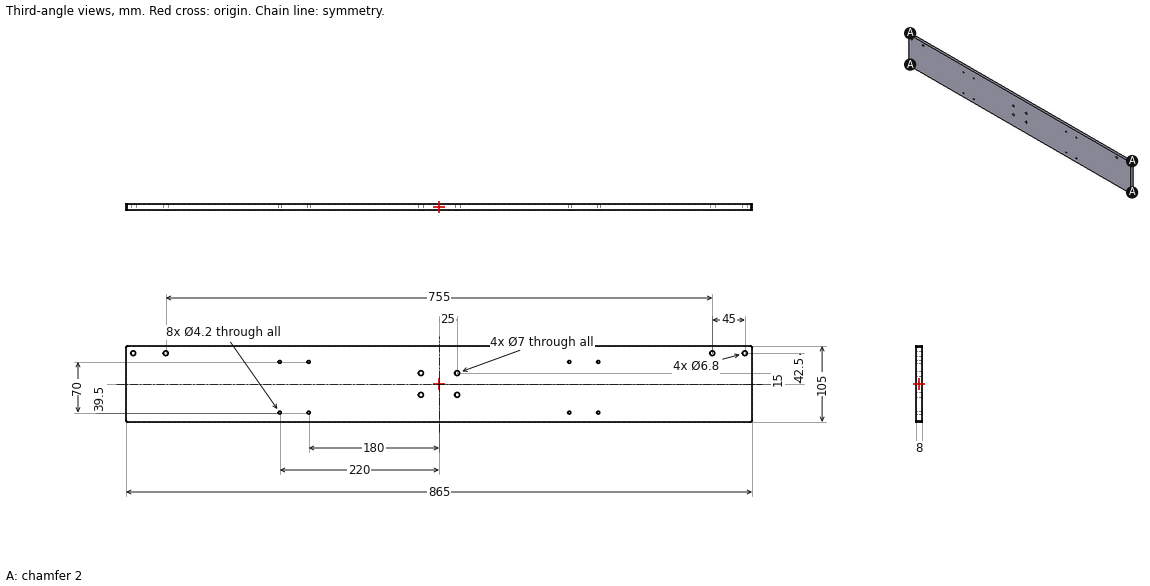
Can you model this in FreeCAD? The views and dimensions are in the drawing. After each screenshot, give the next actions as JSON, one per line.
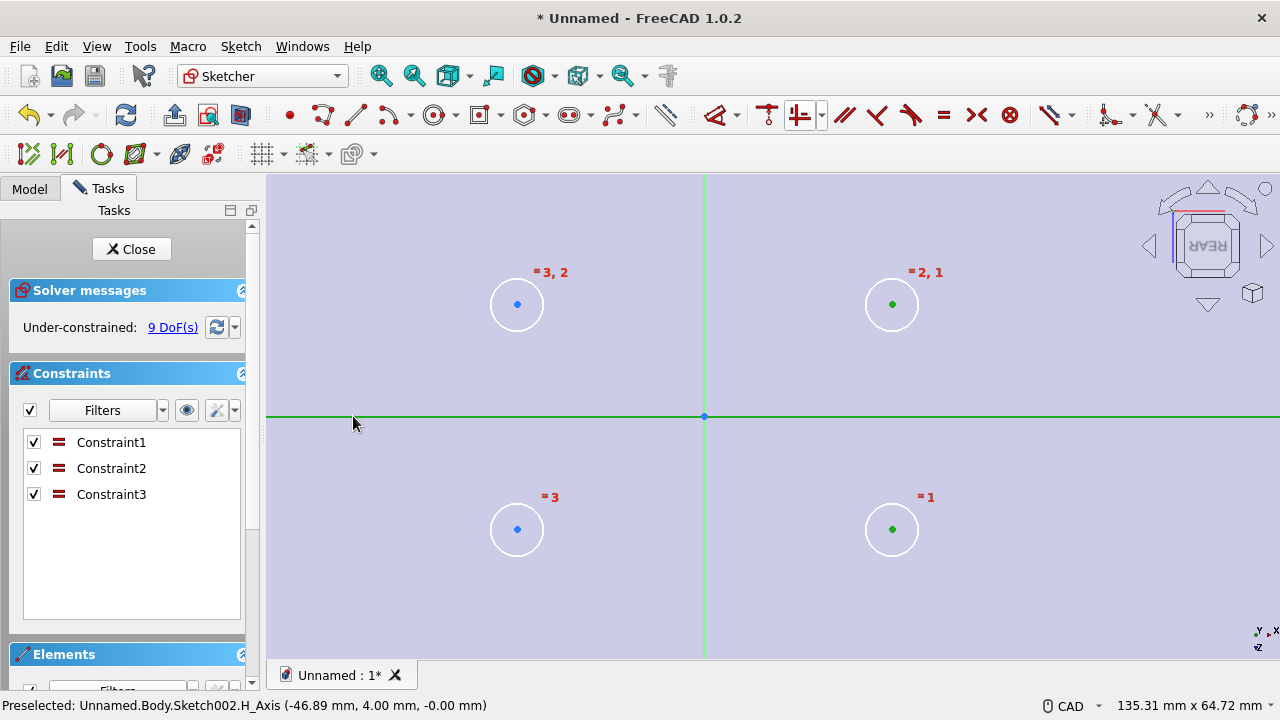
{"action": "key", "text": "s"}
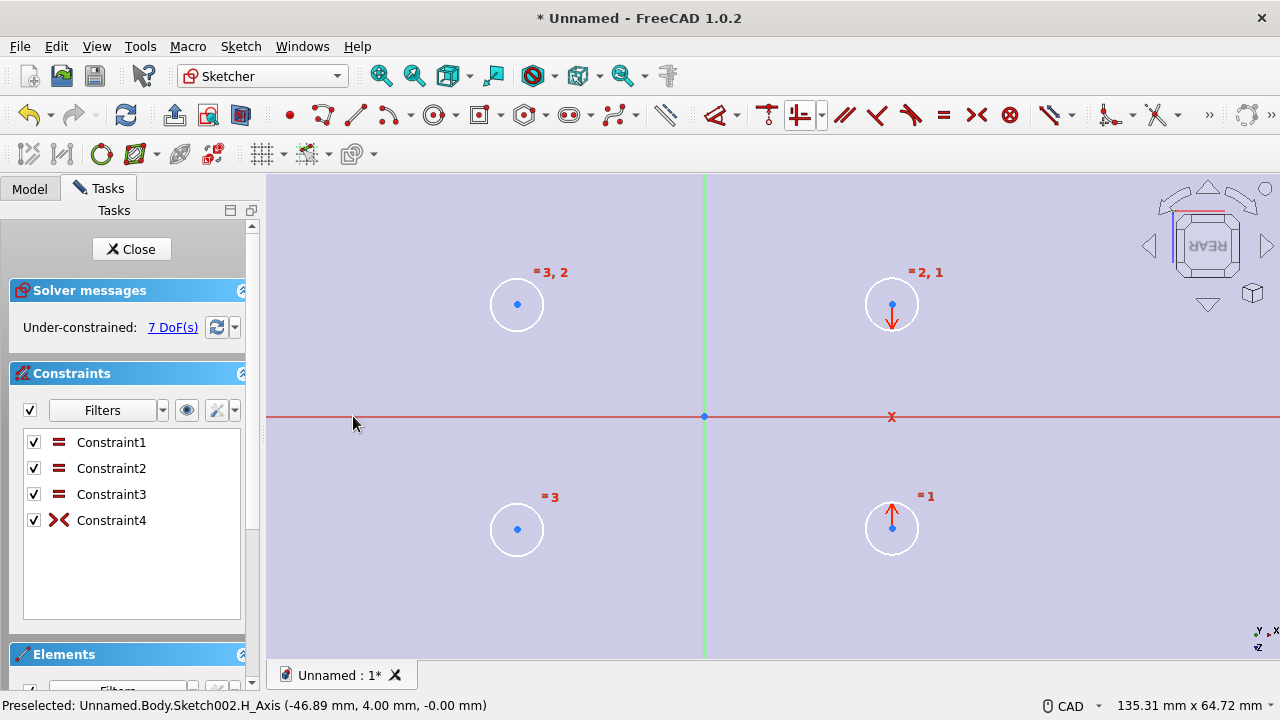
{"action": "left_click", "coordinate": [892, 304]}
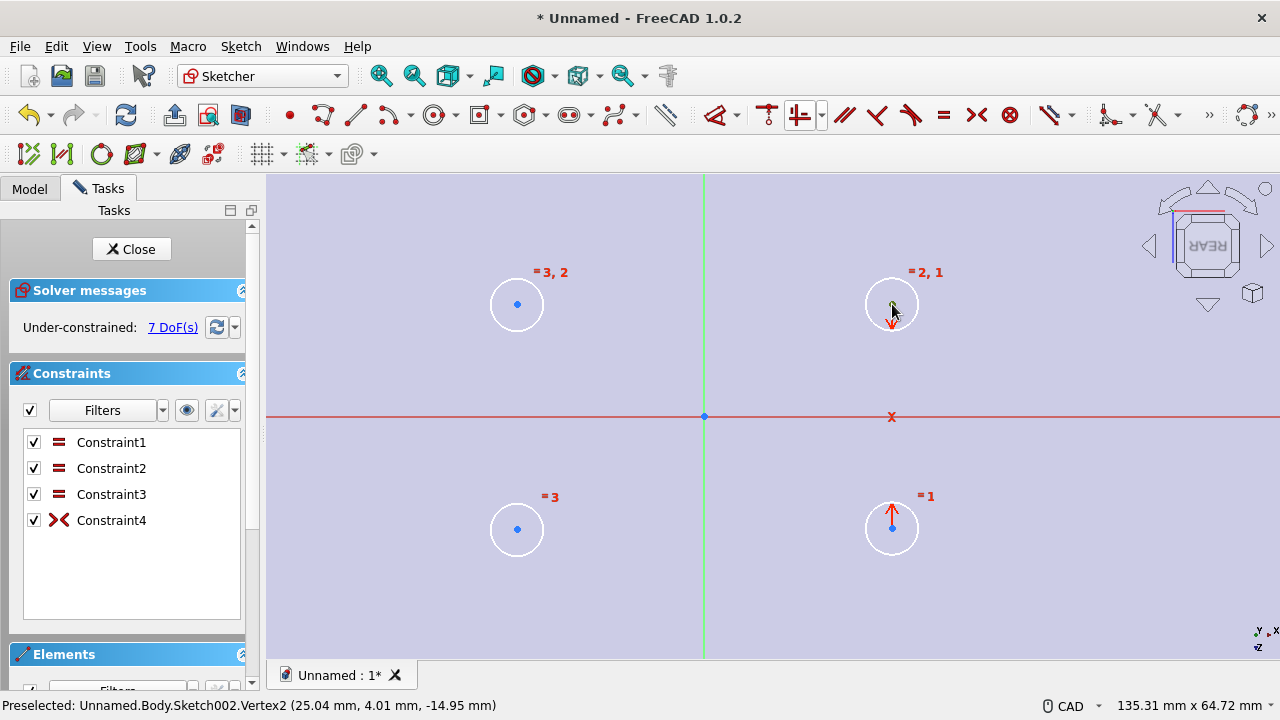
{"action": "left_click", "coordinate": [517, 305]}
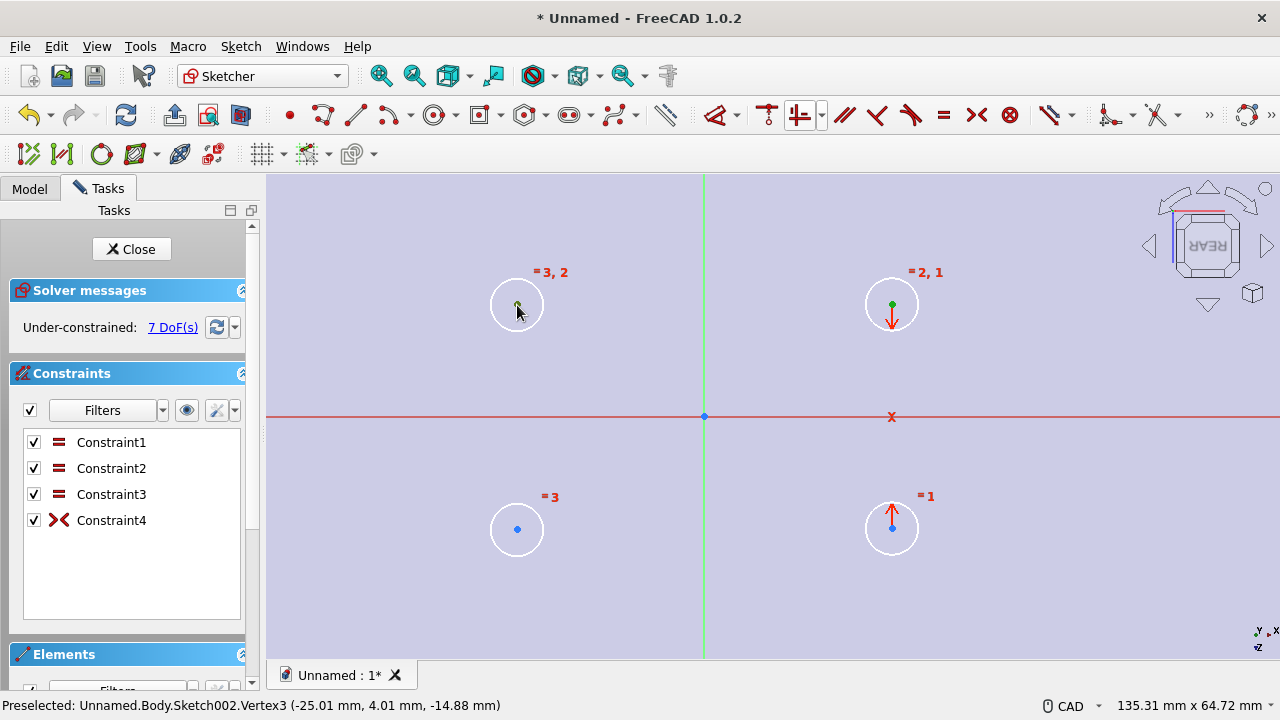
{"action": "left_click", "coordinate": [704, 600]}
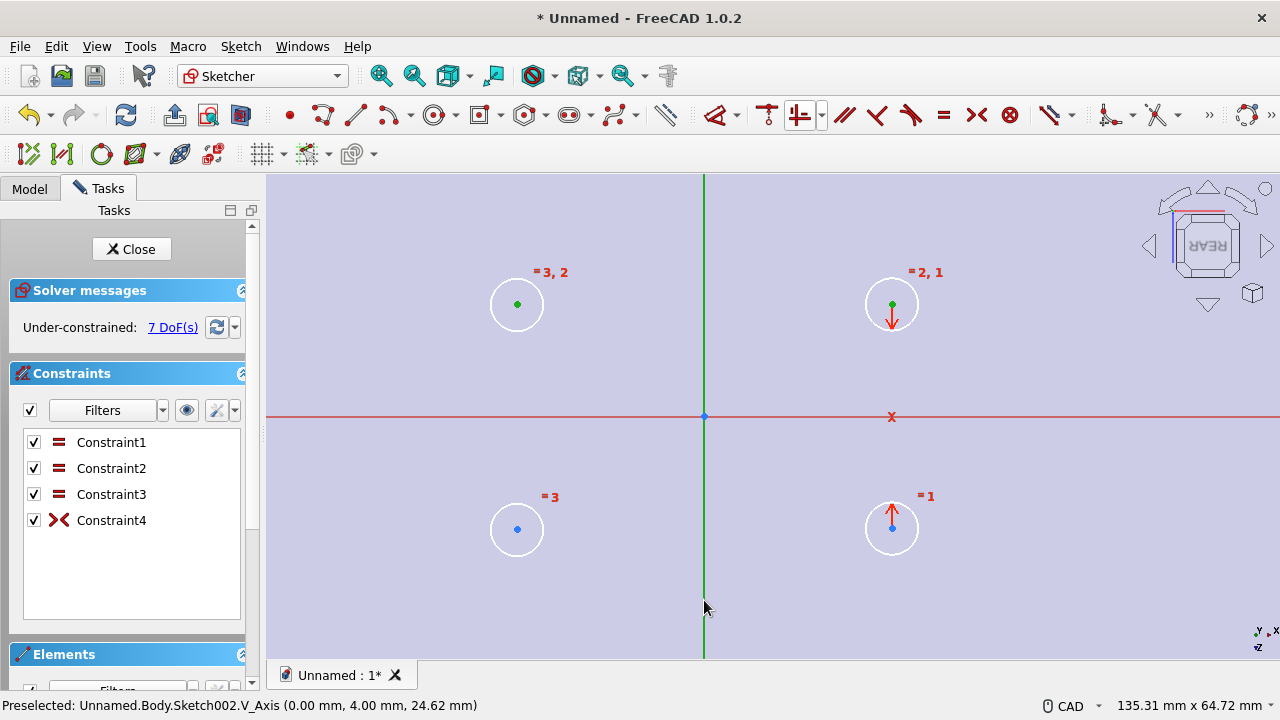
{"action": "key", "text": "s"}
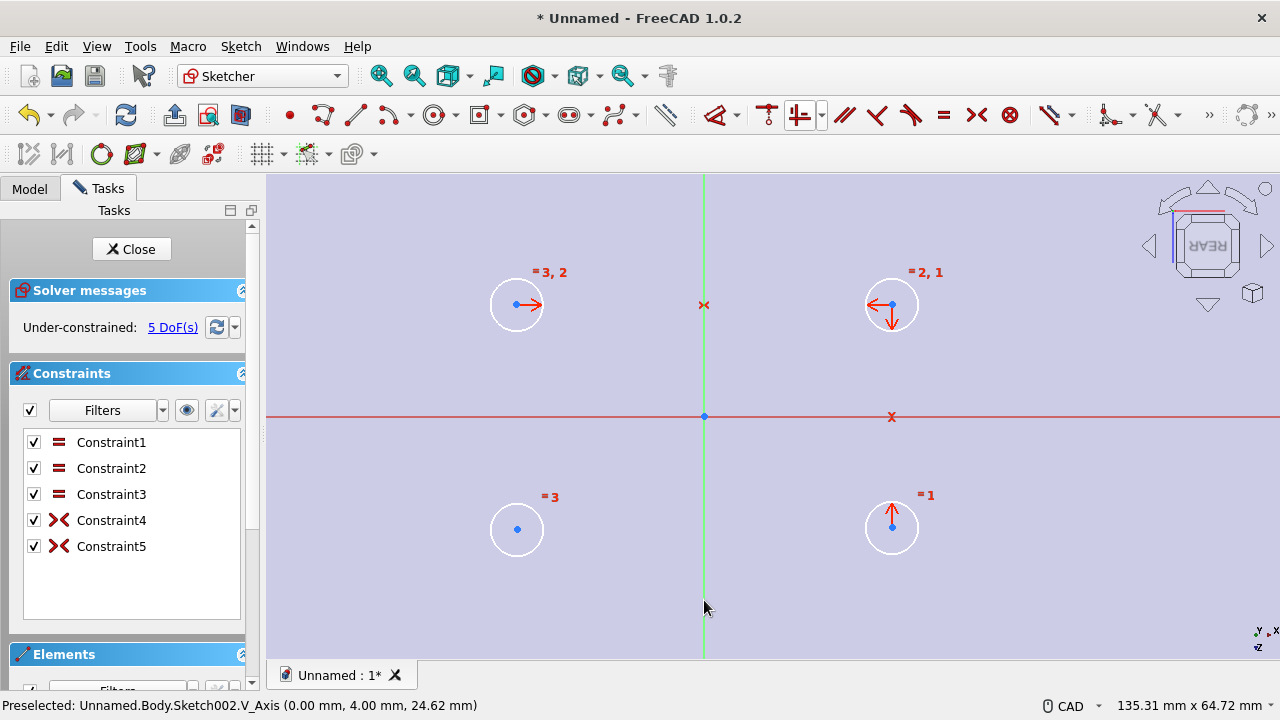
{"action": "left_click", "coordinate": [892, 528]}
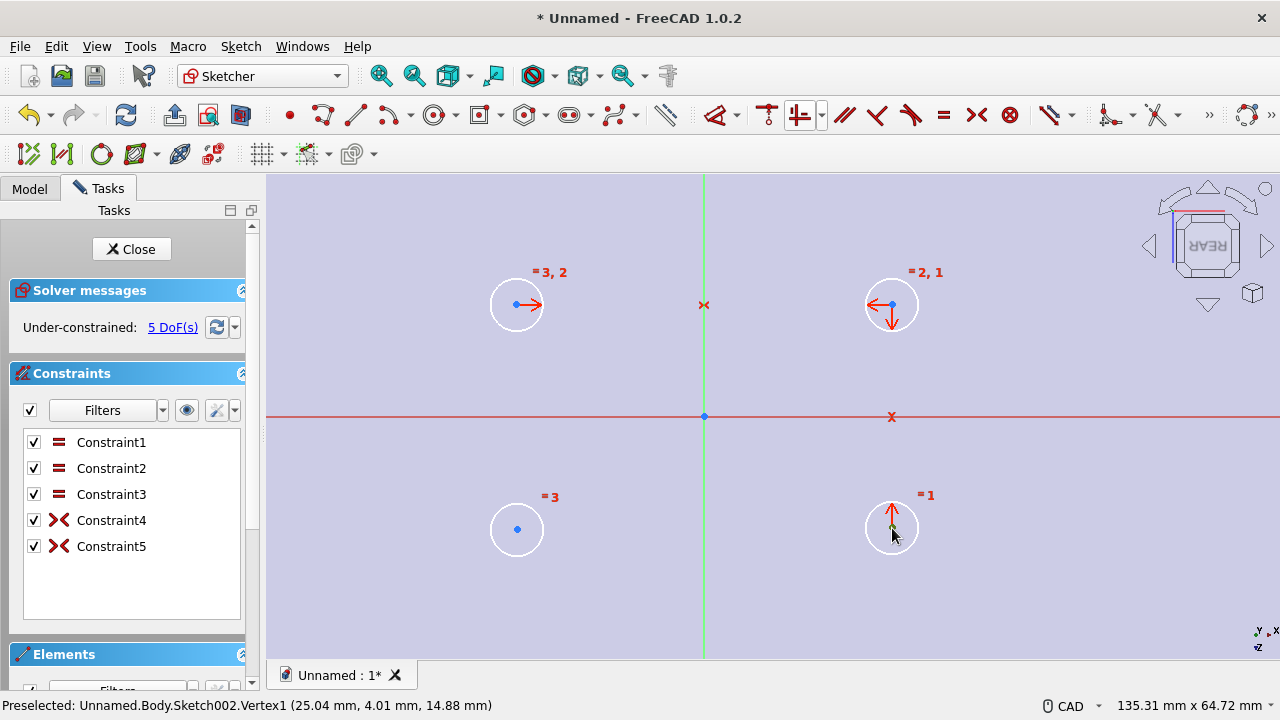
{"action": "left_click", "coordinate": [517, 530]}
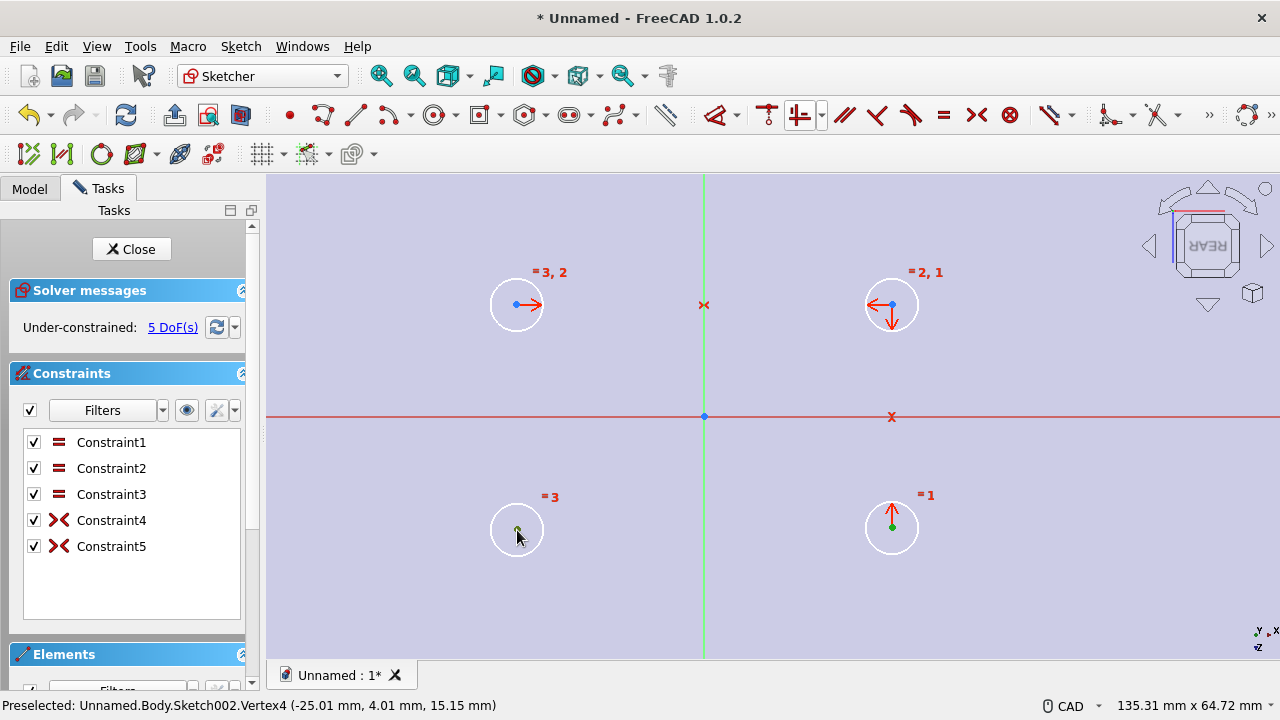
{"action": "left_click", "coordinate": [704, 600]}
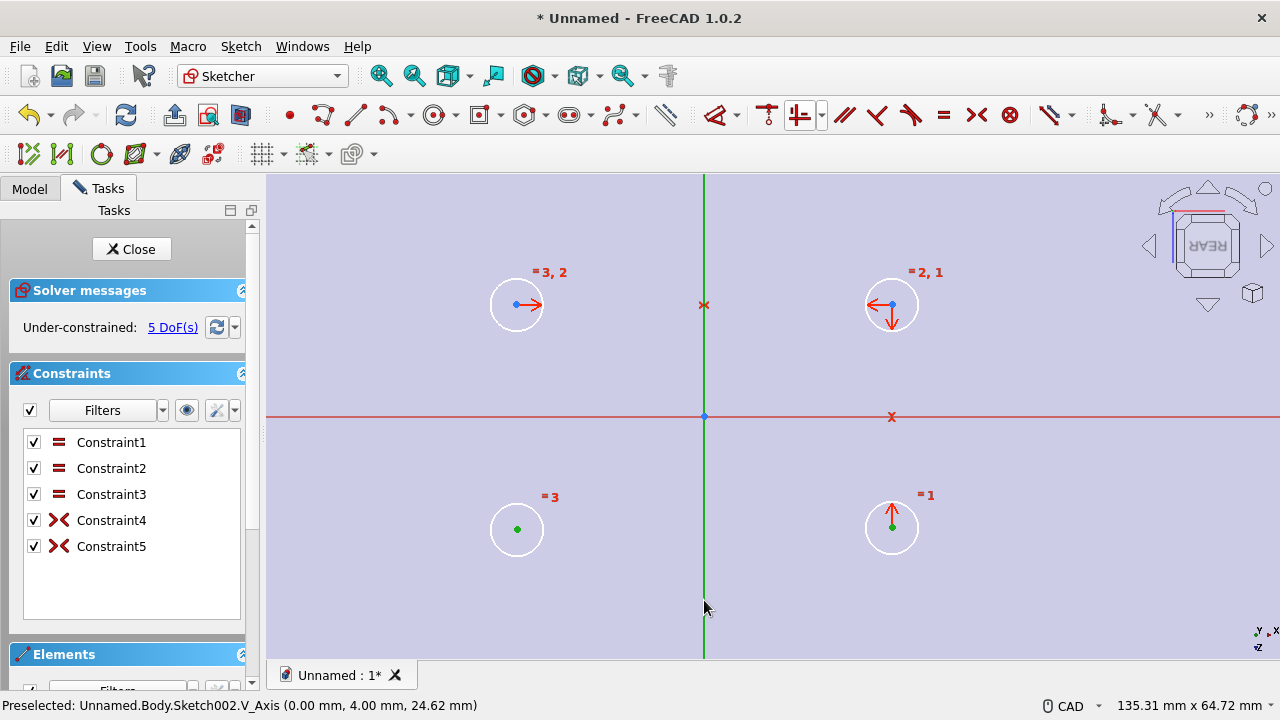
{"action": "key", "text": "s"}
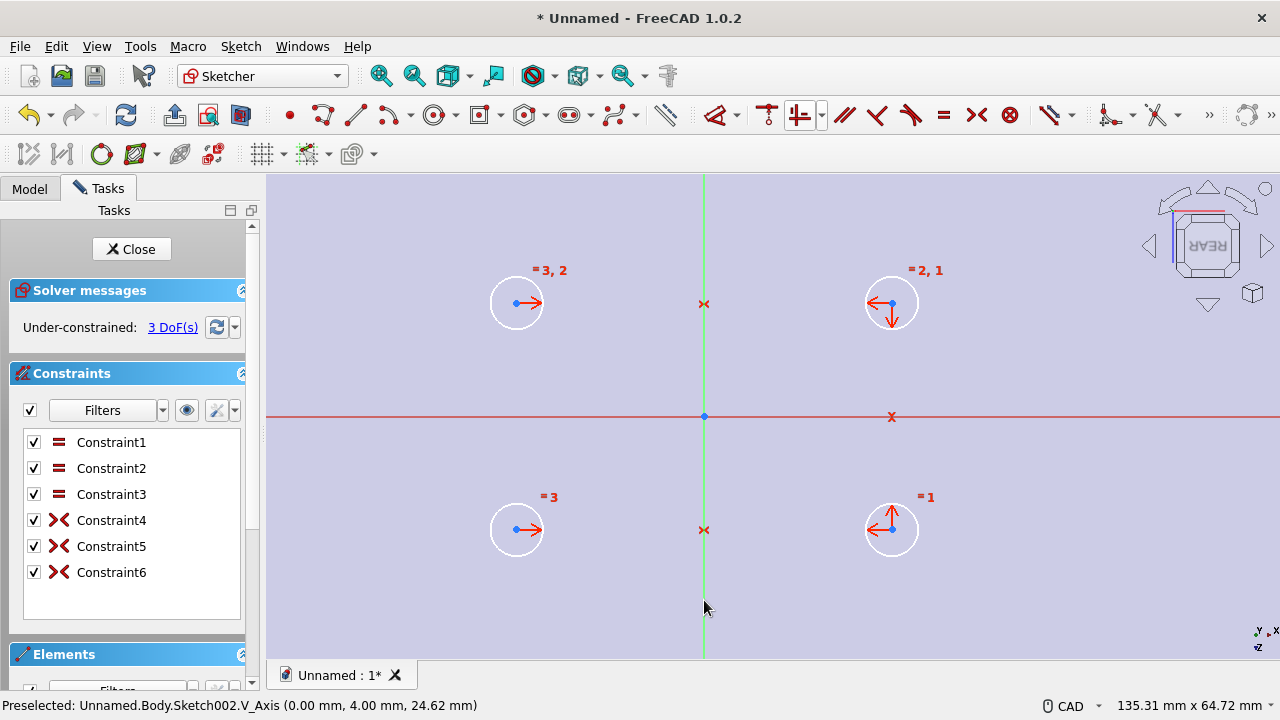
{"action": "left_click", "coordinate": [714, 116]}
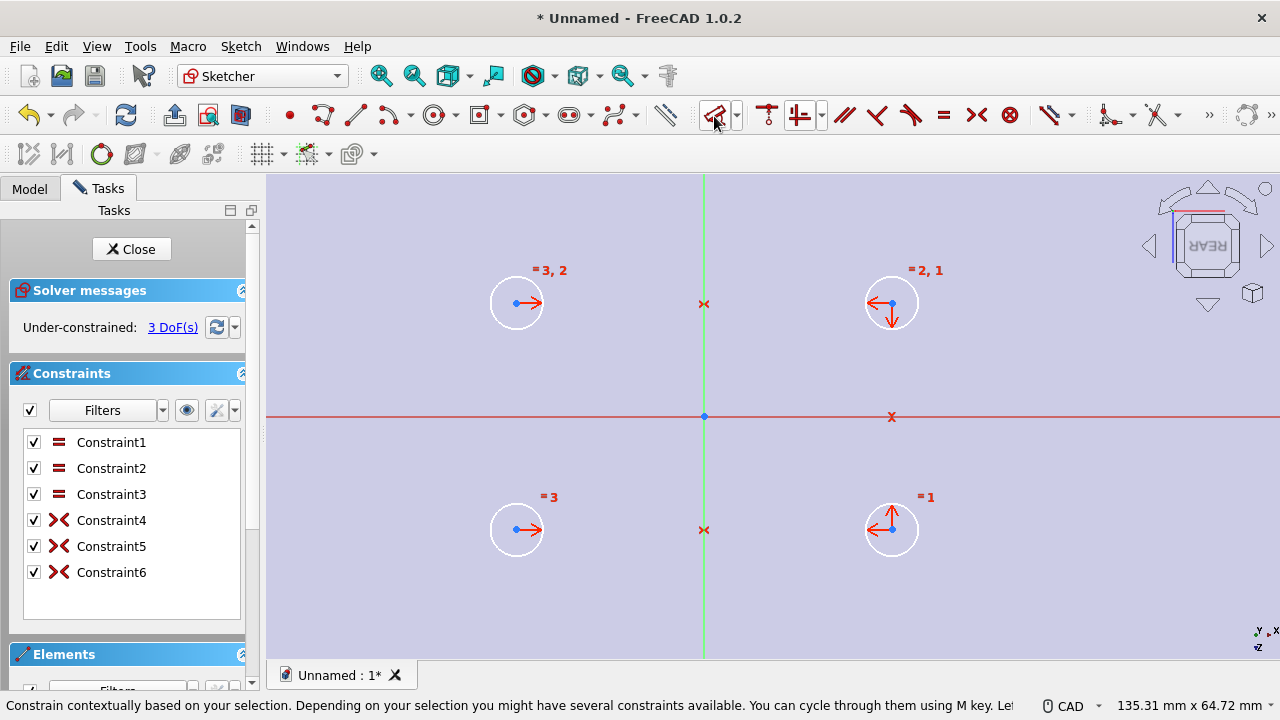
{"action": "left_click", "coordinate": [910, 511]}
{"action": "left_click", "coordinate": [932, 488]}